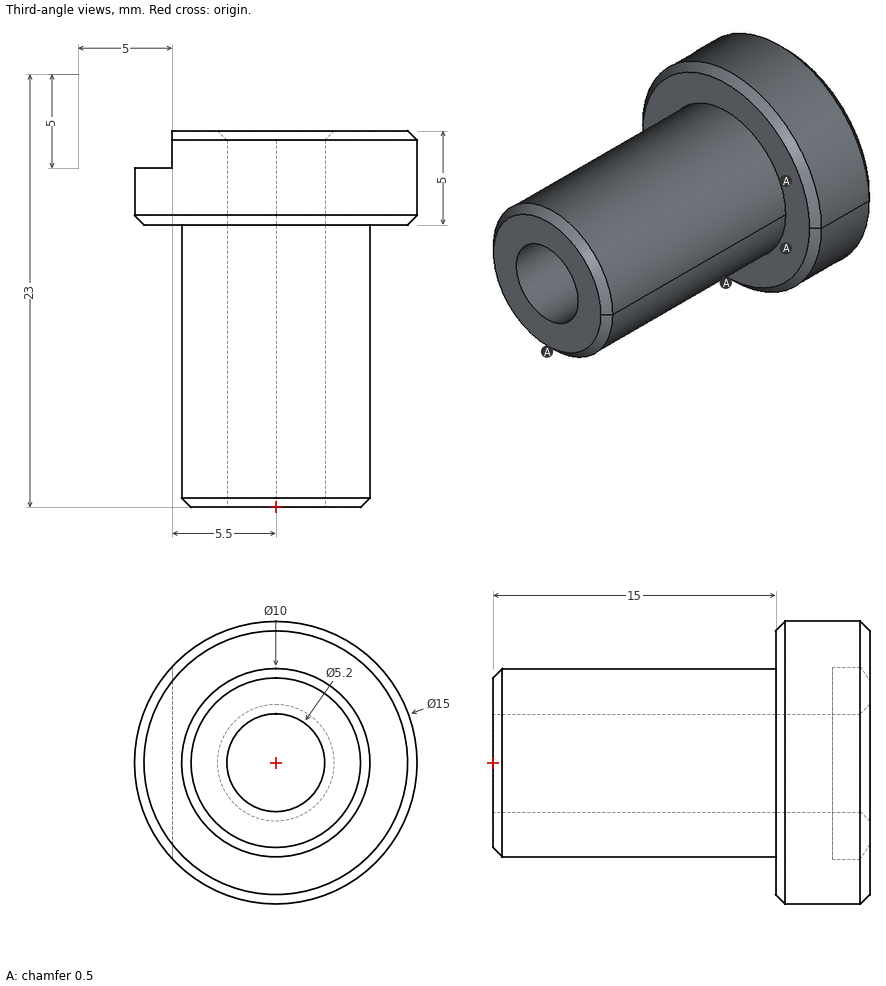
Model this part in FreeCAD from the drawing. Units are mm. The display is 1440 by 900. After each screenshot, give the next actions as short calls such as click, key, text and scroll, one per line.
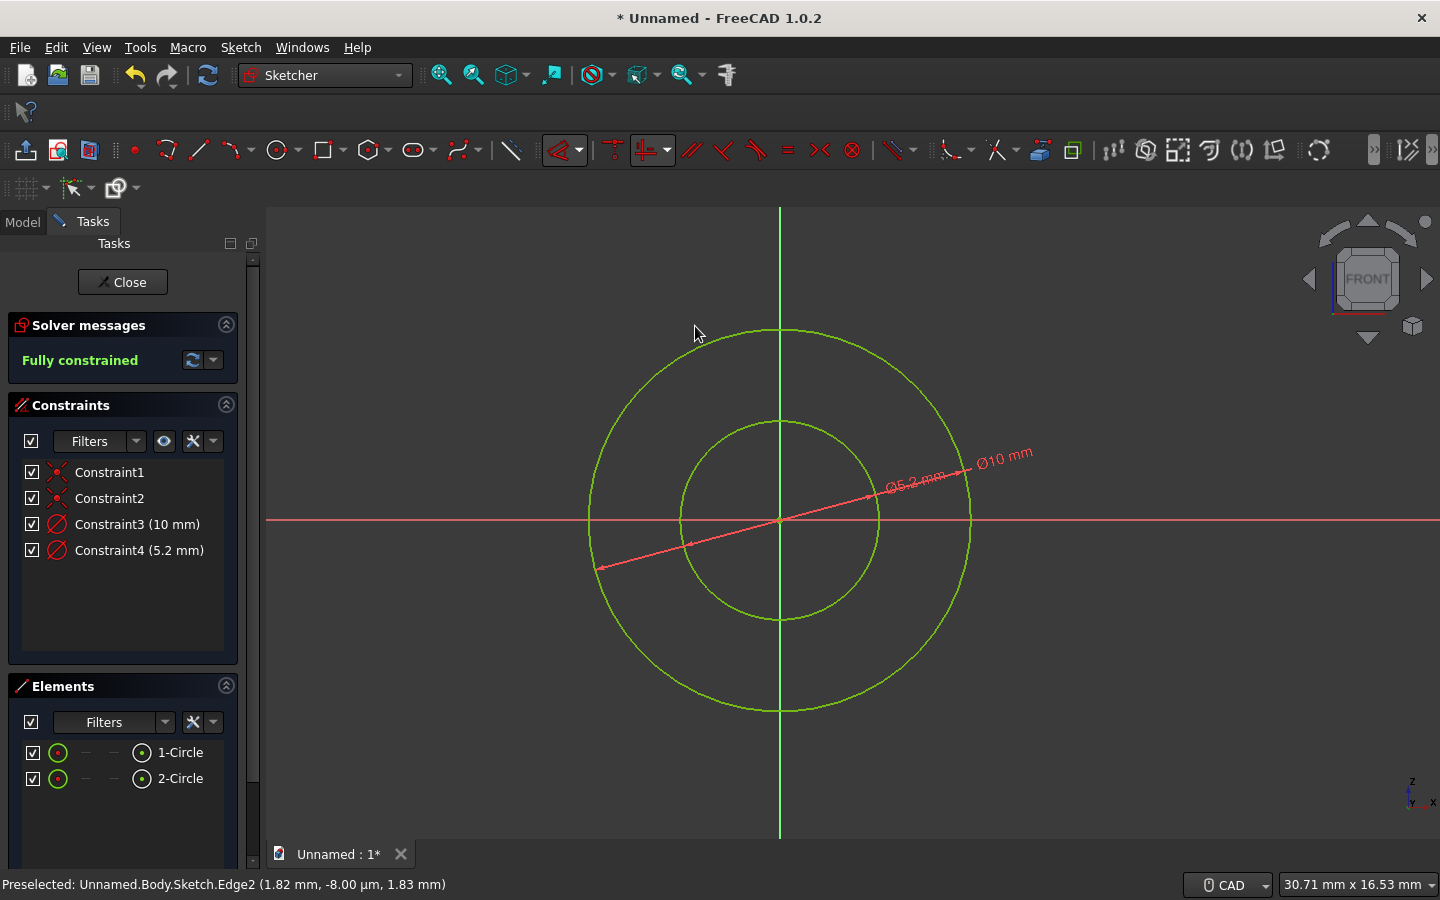
click(123, 282)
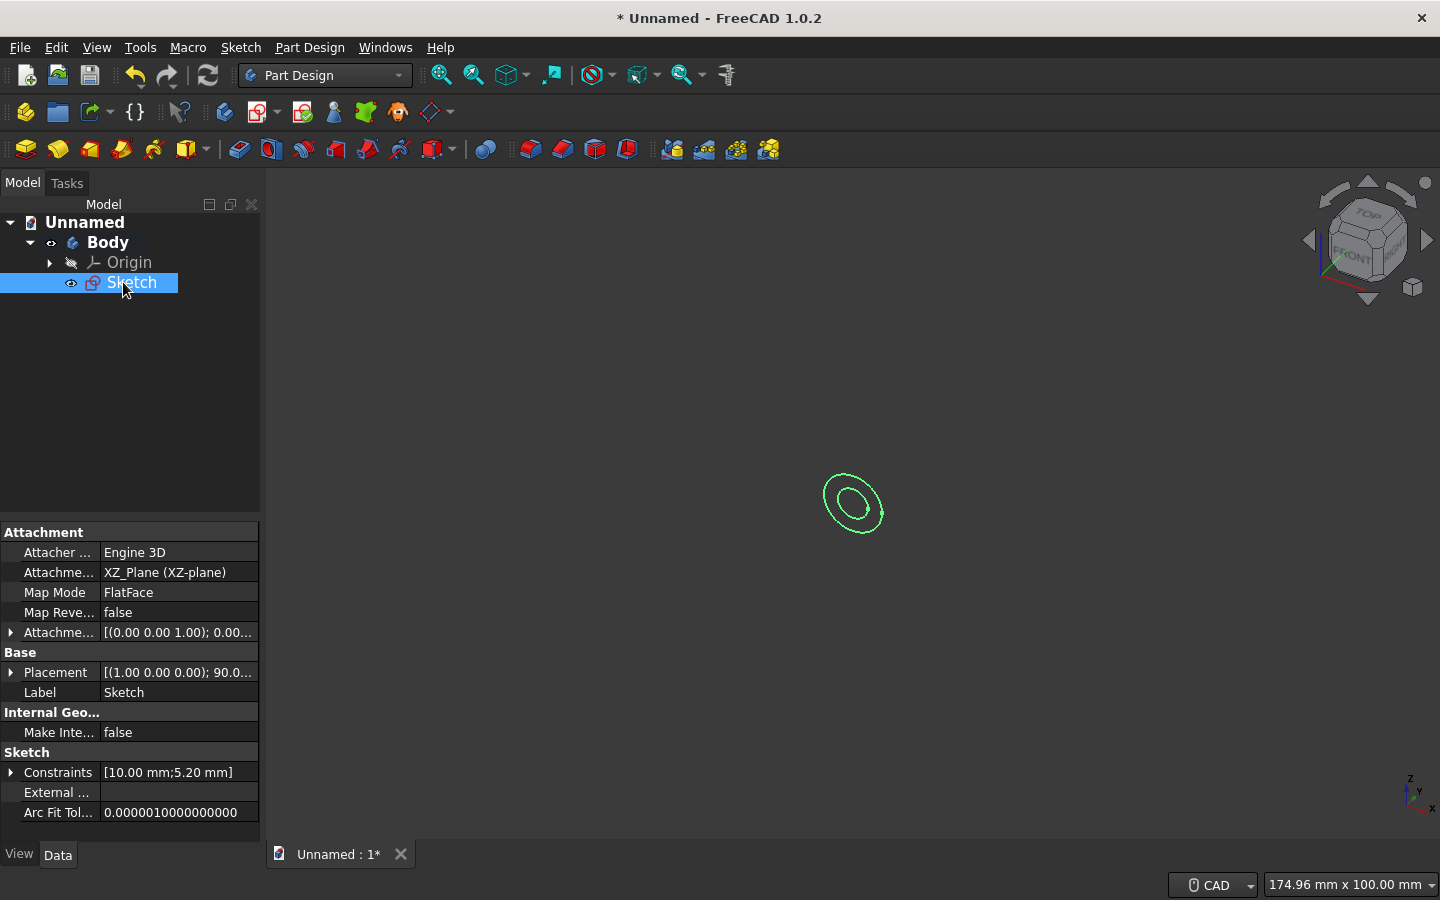
click(26, 150)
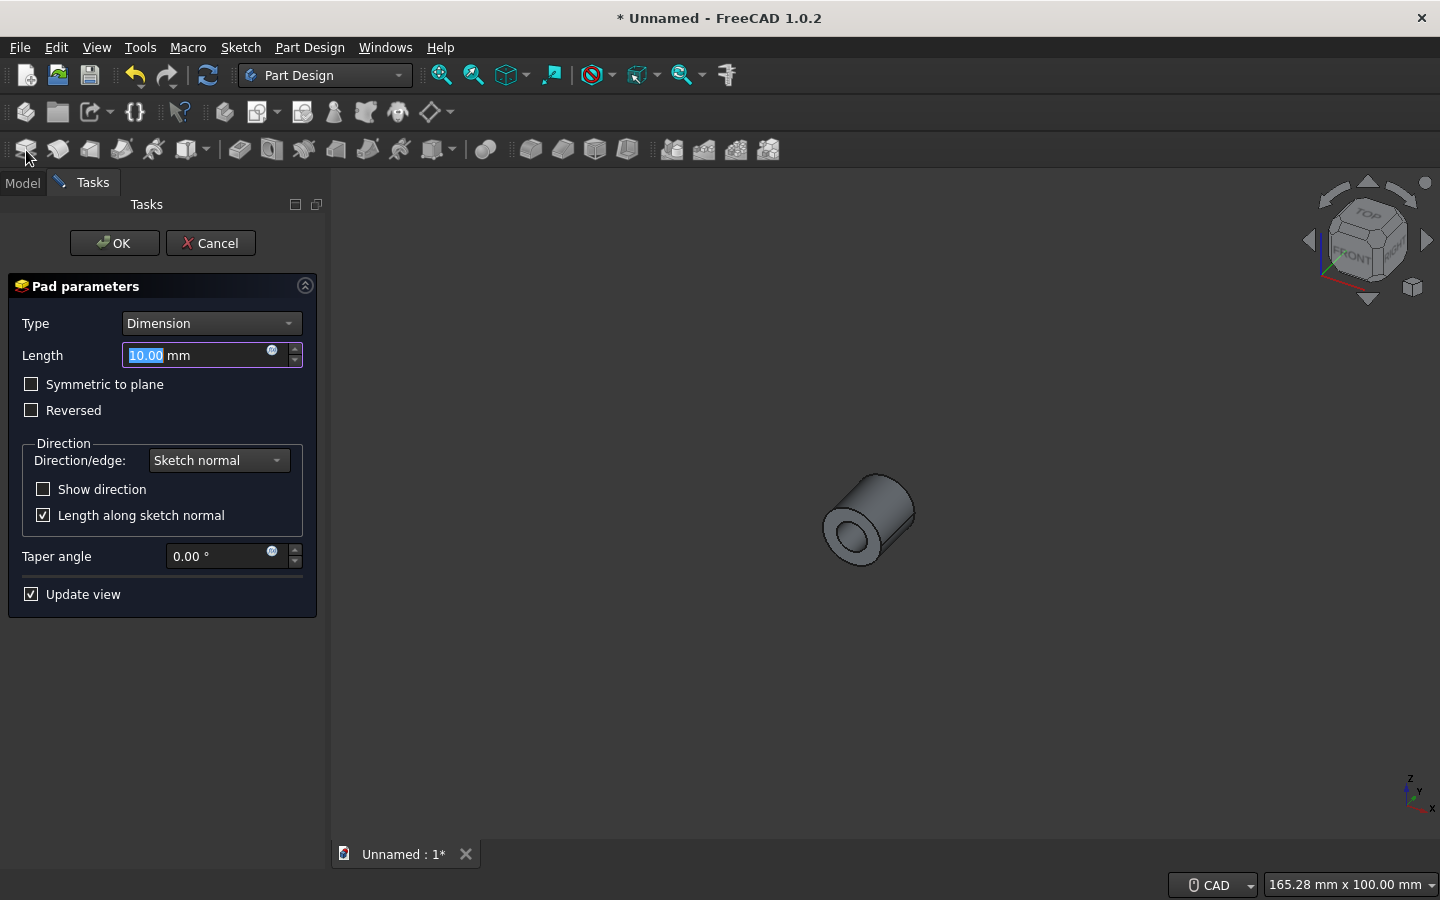
text(15)
key(Tab)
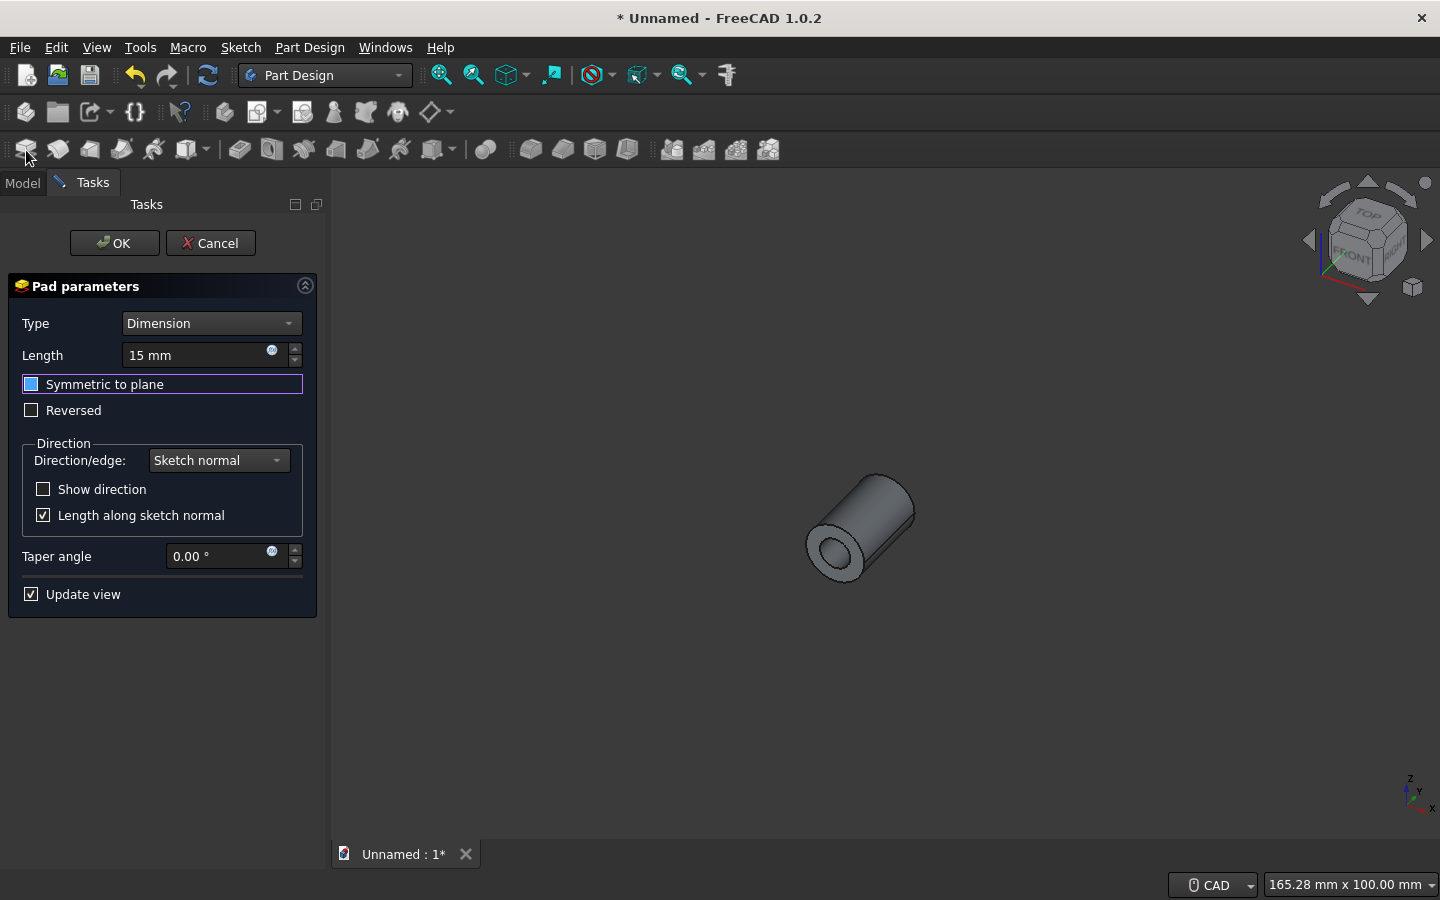
click(30, 410)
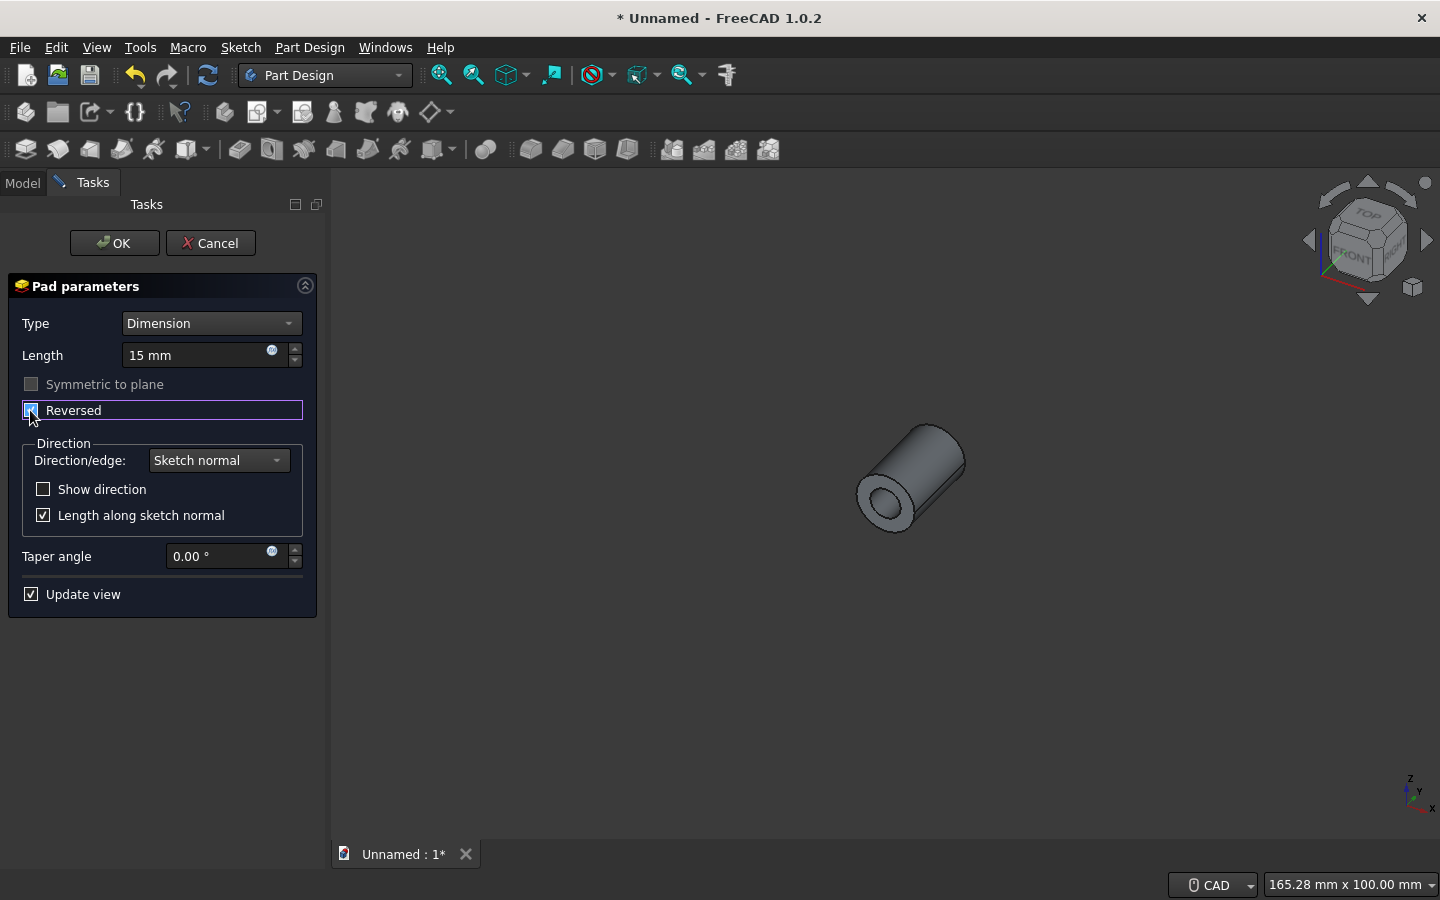
click(115, 243)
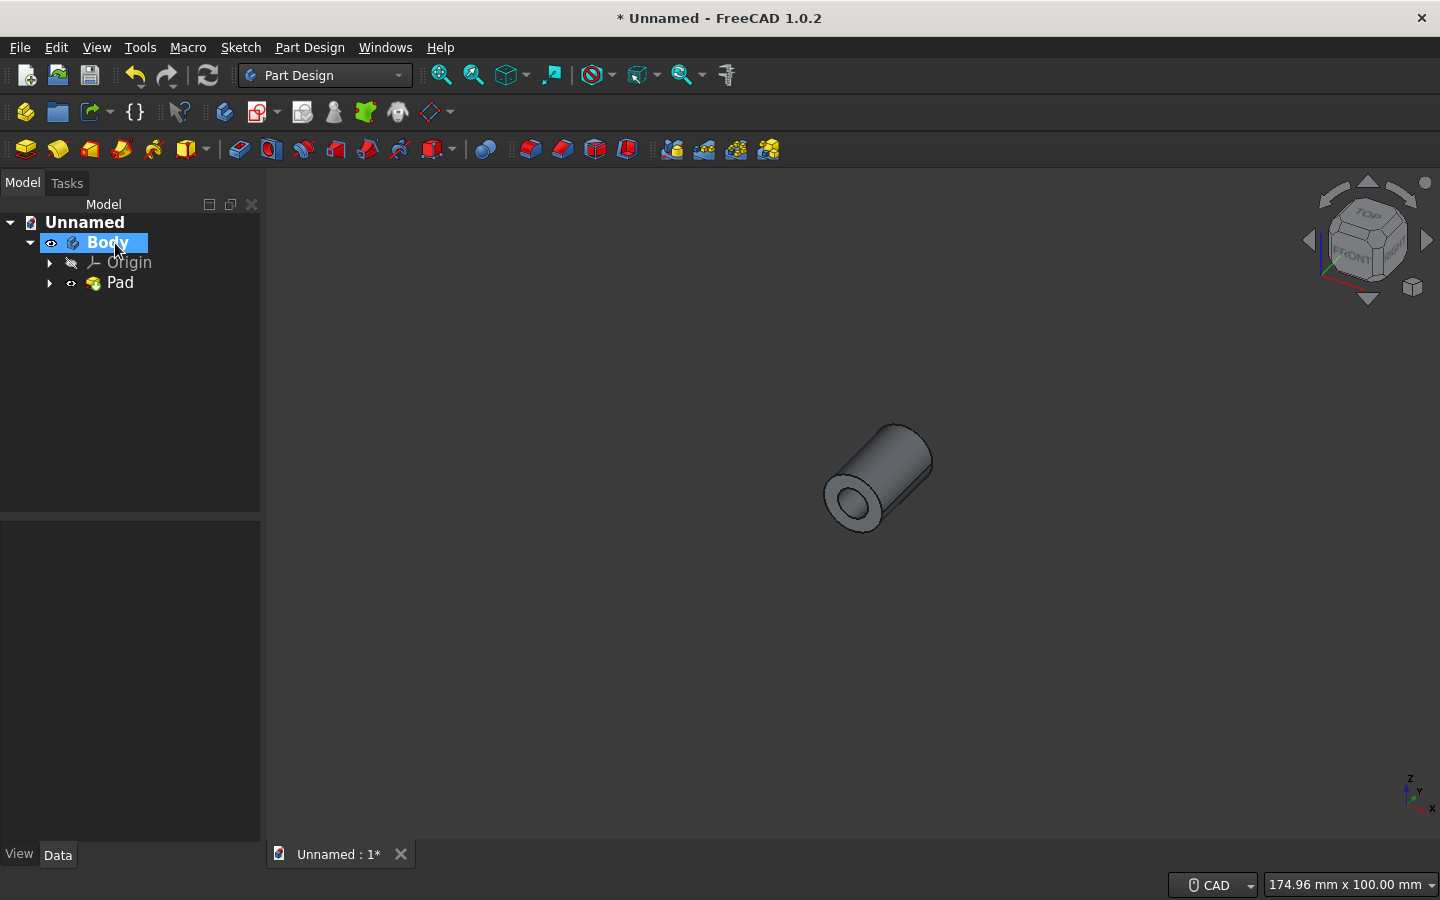
click(442, 76)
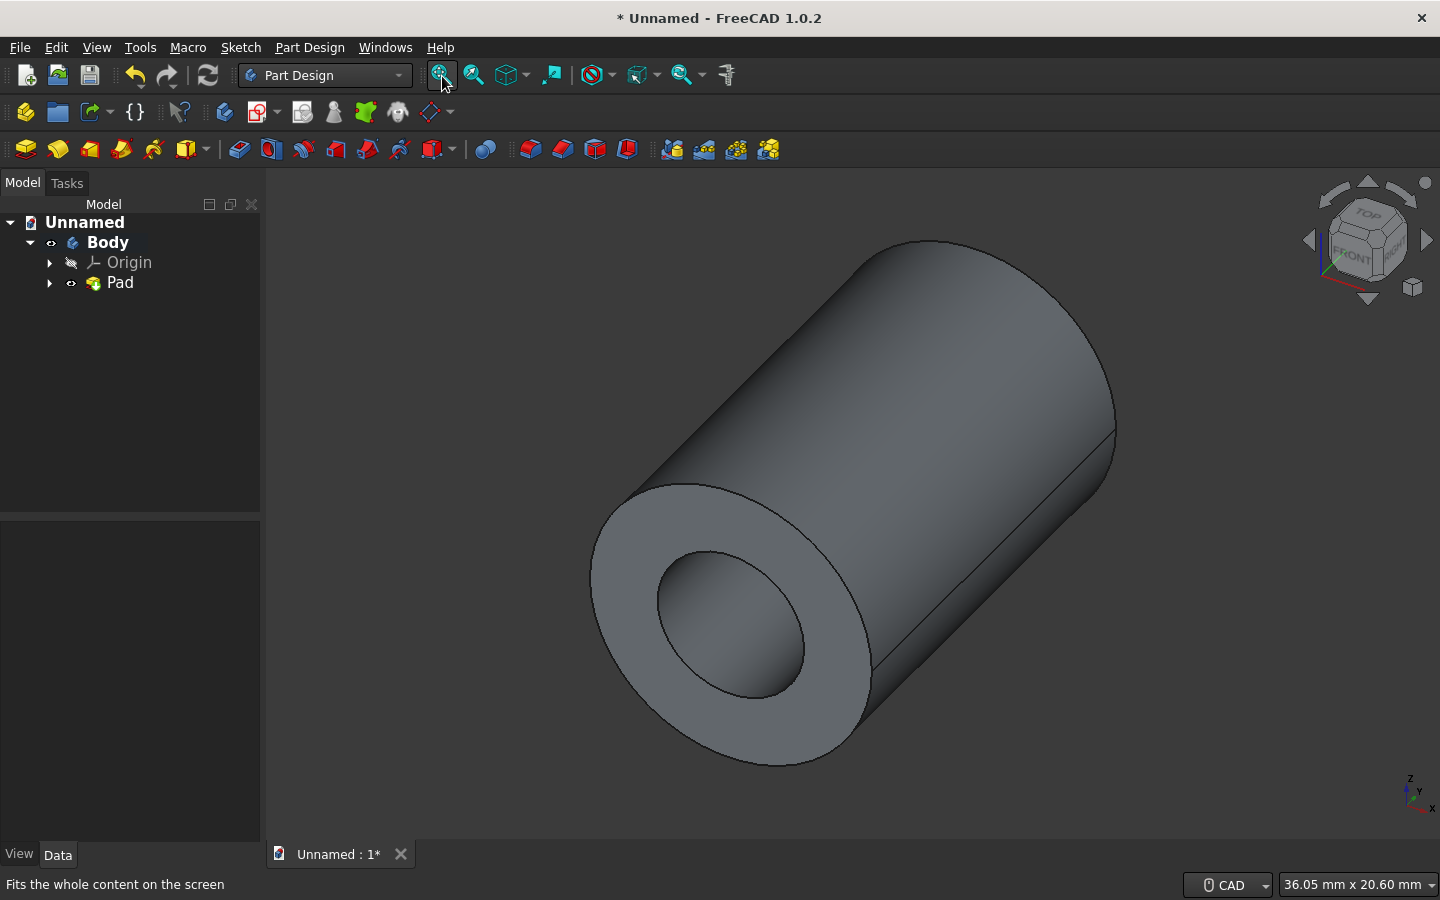
key(4)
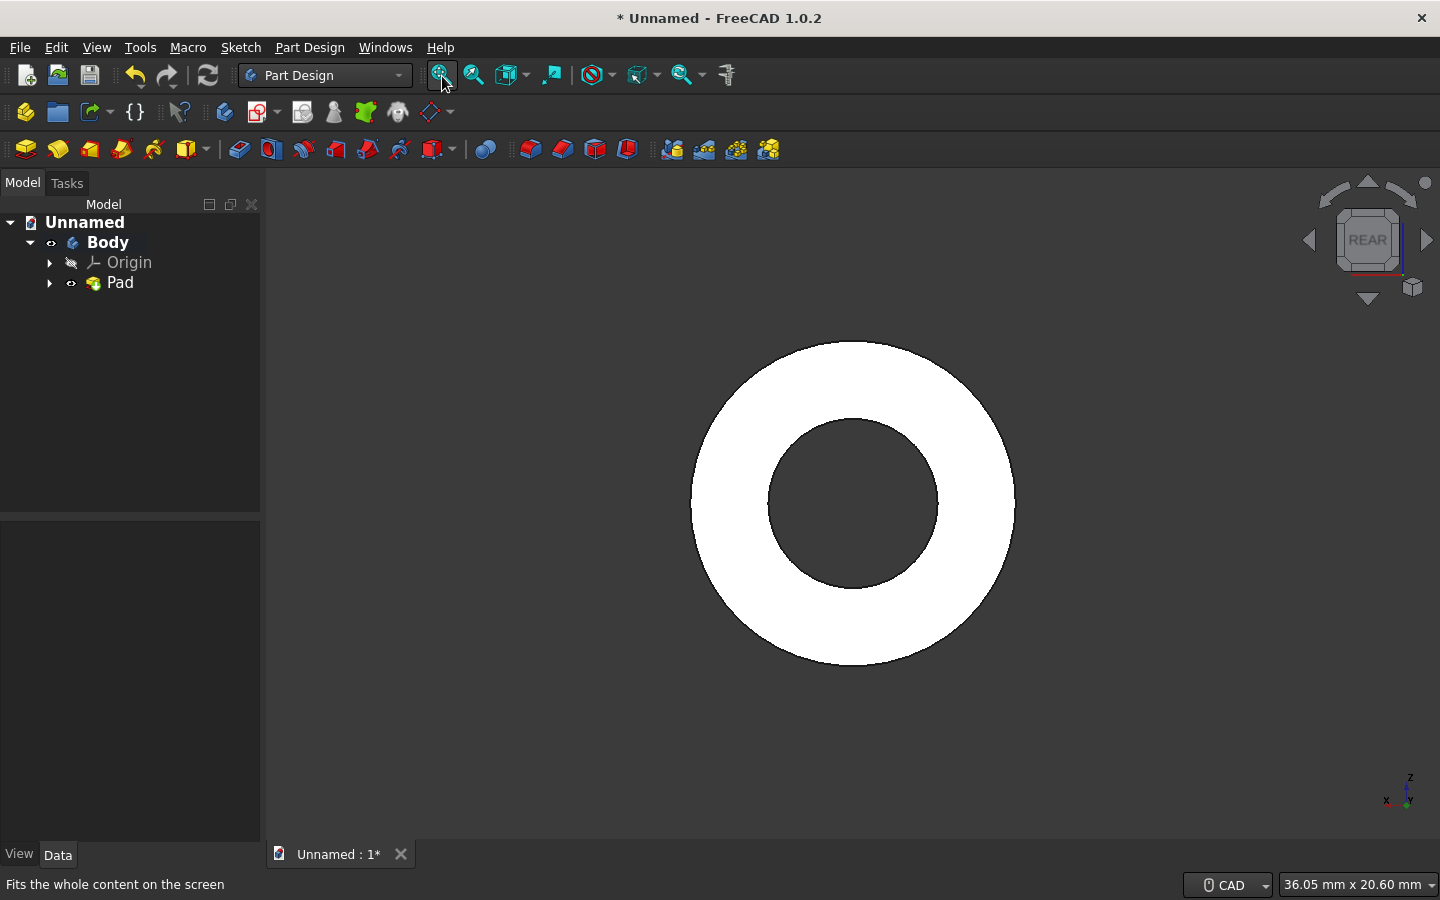
click(760, 596)